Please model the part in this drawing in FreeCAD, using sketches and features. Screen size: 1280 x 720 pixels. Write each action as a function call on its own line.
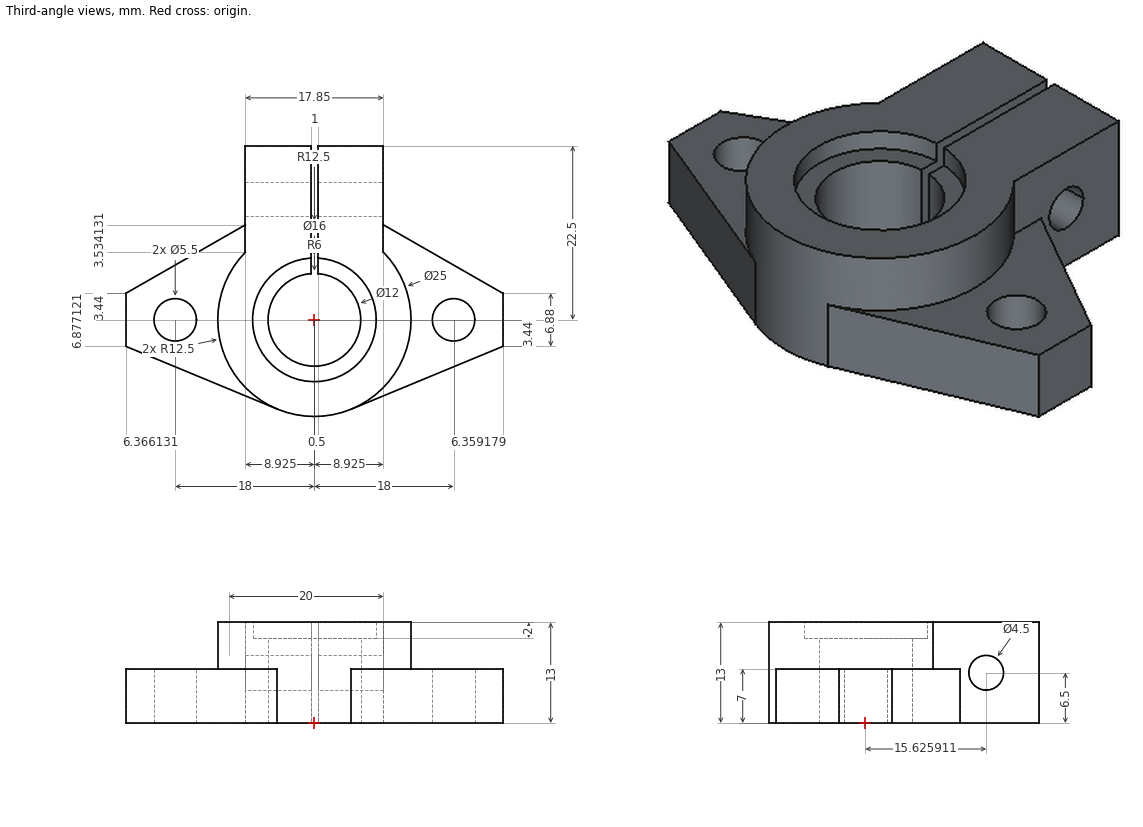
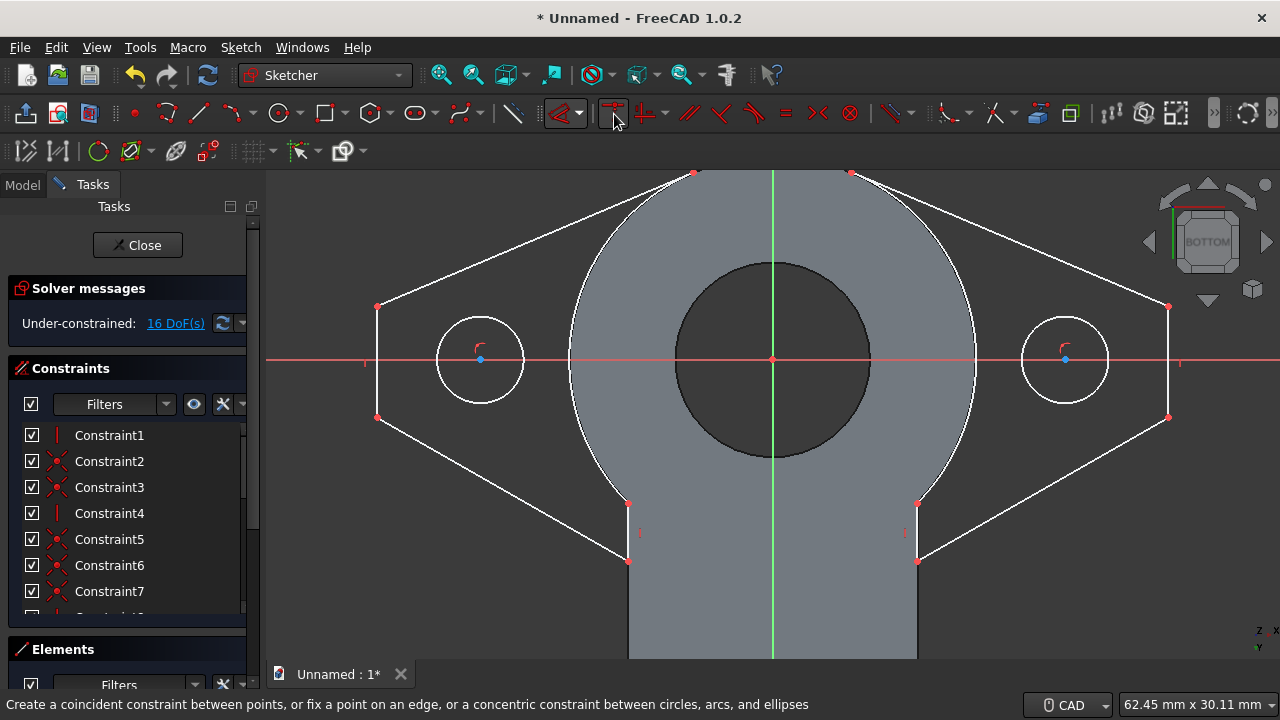
click(603, 247)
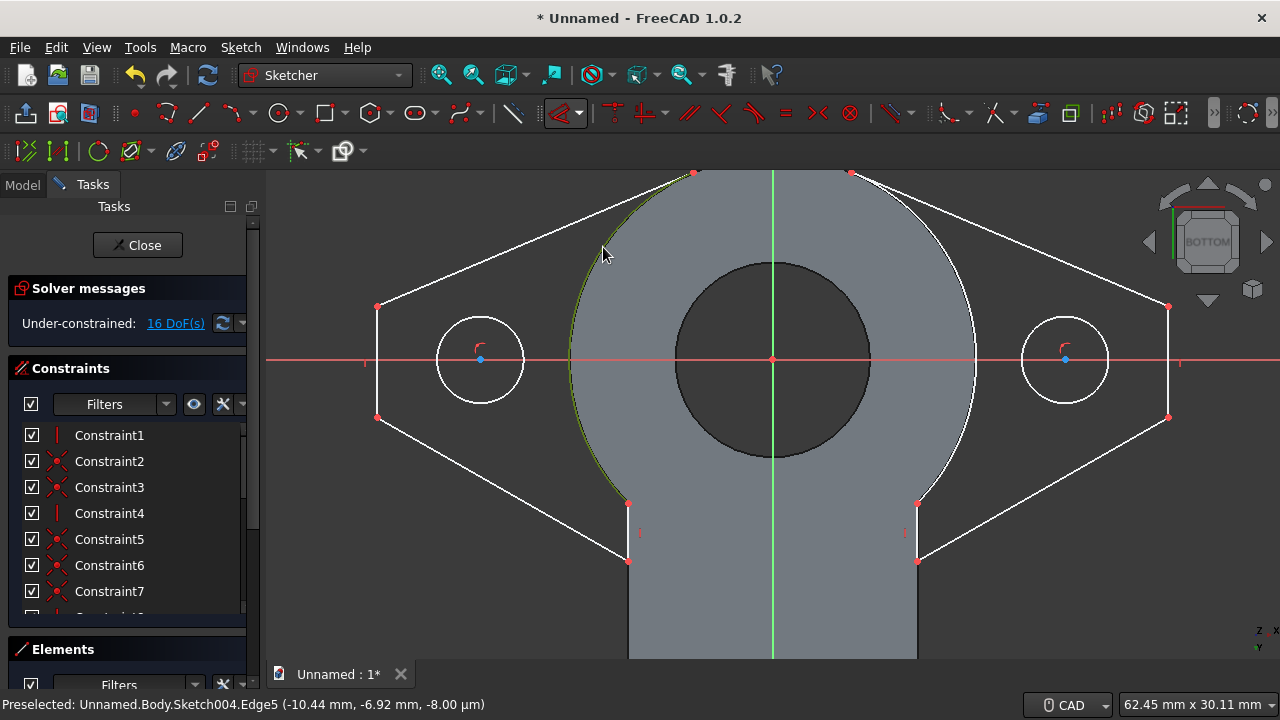
click(972, 399)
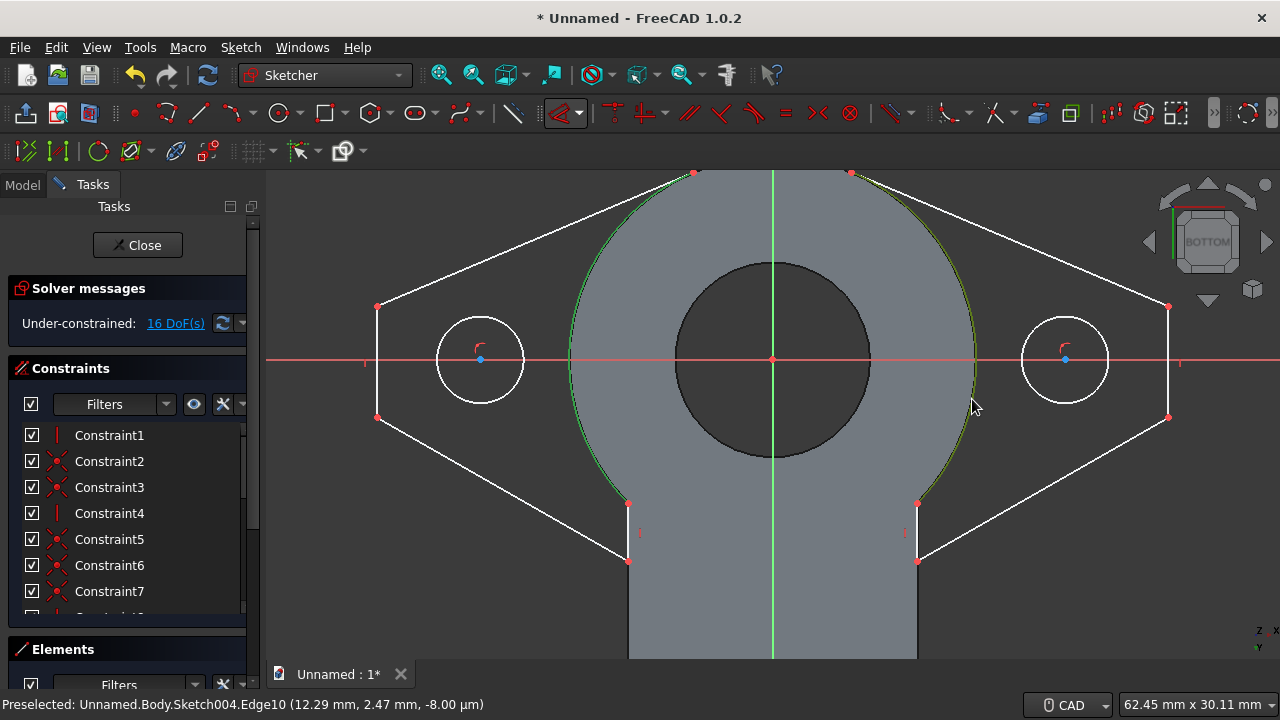
click(786, 114)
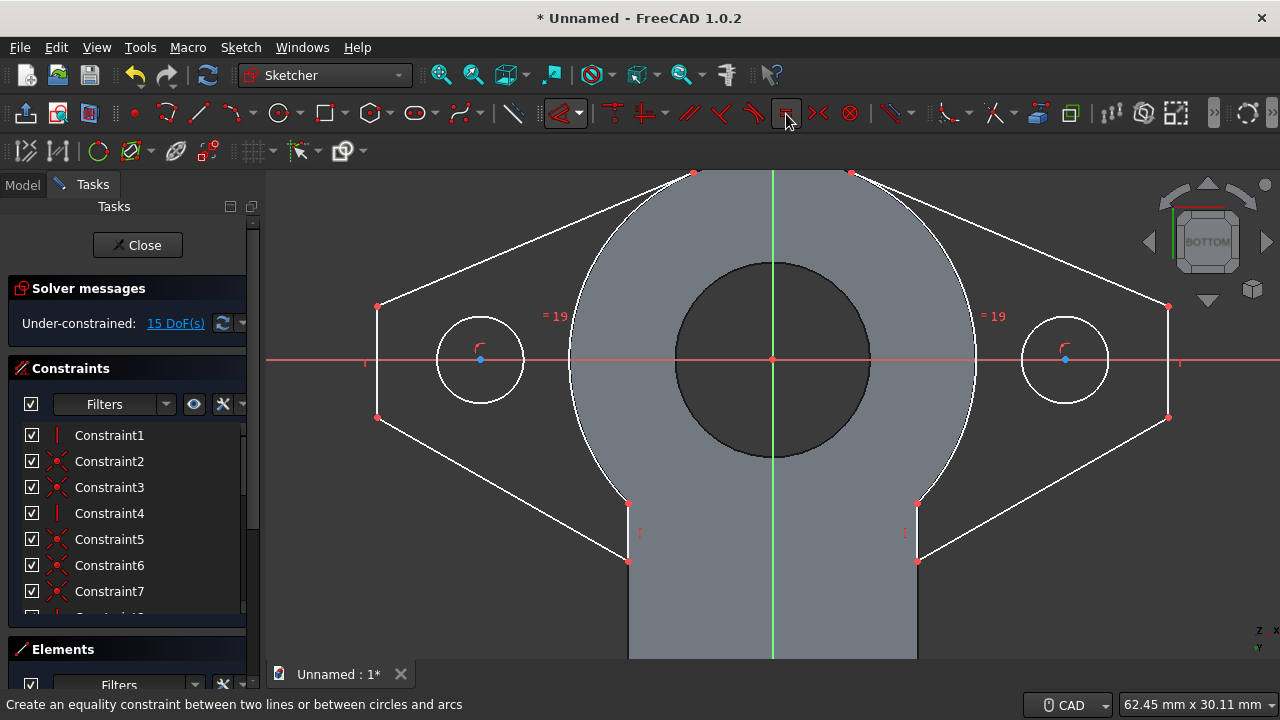
click(511, 329)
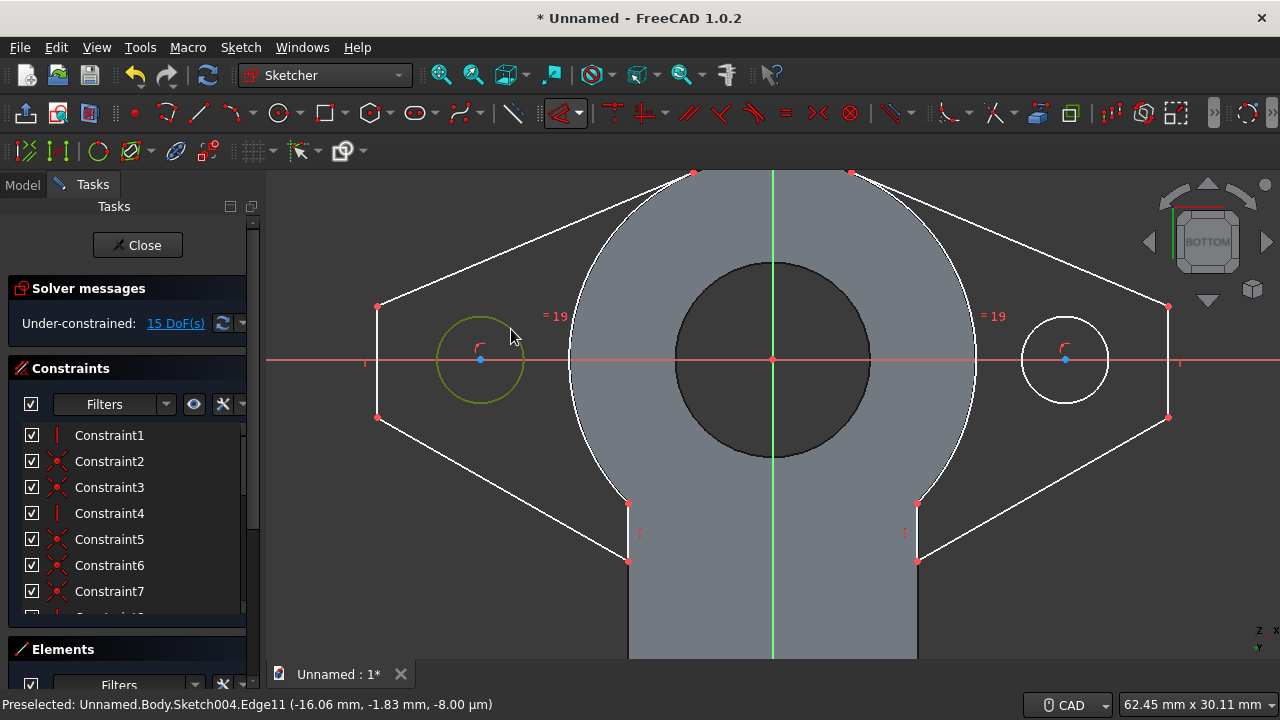
click(1096, 329)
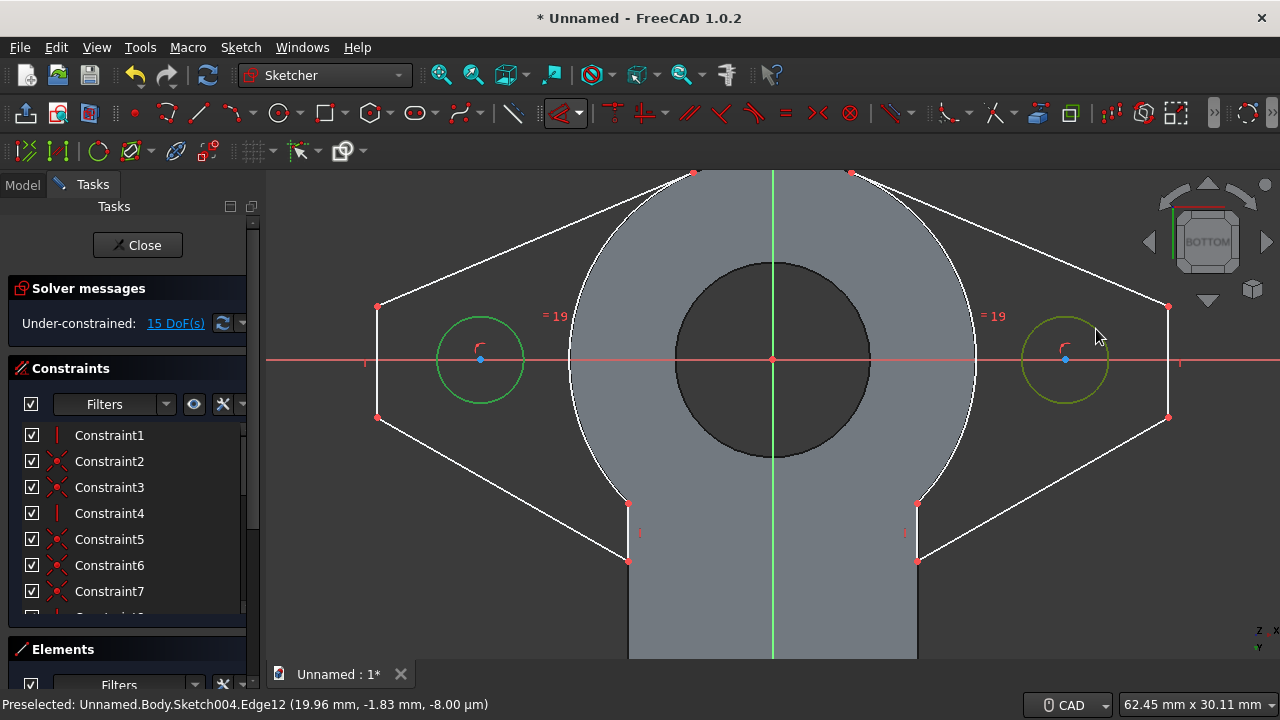
click(786, 114)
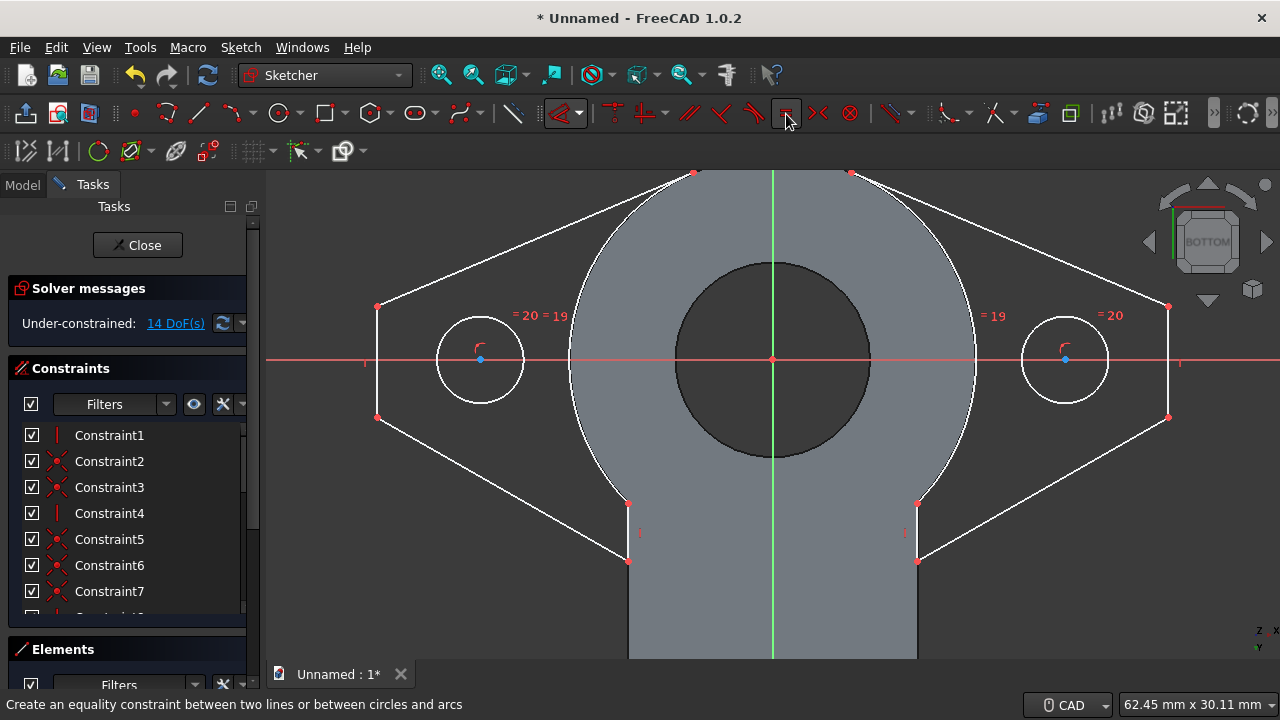
click(603, 247)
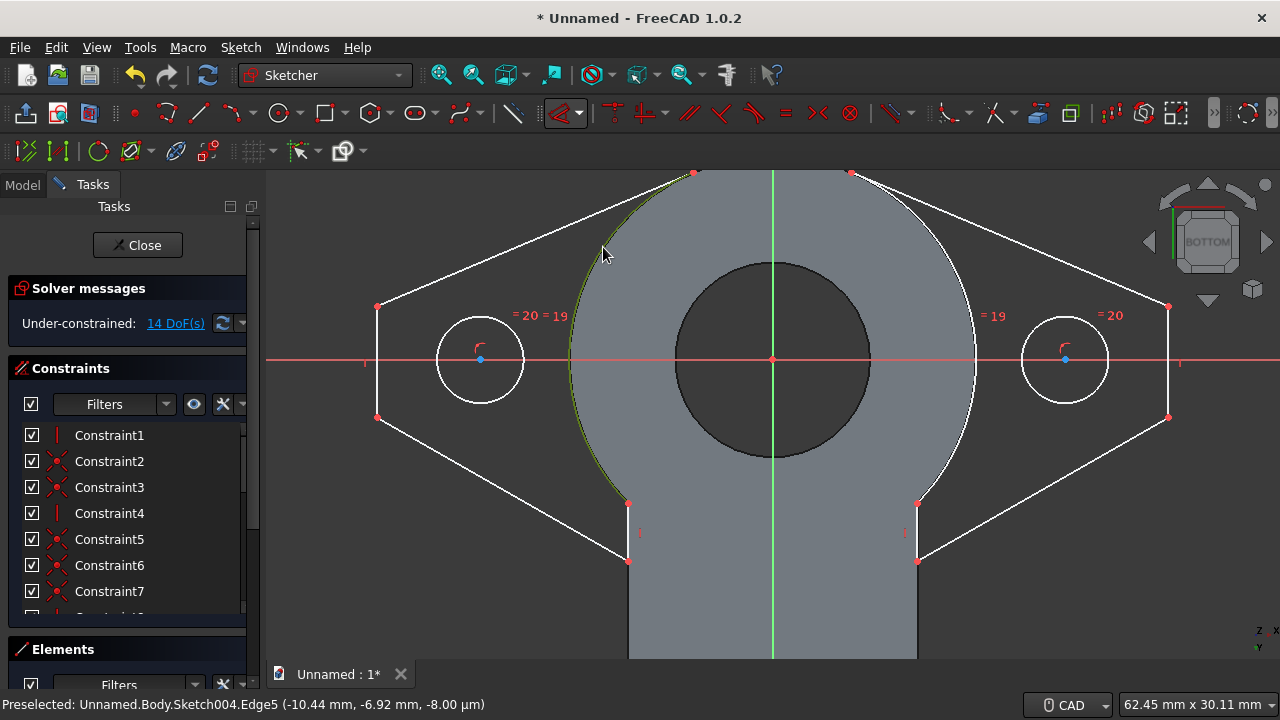
click(582, 114)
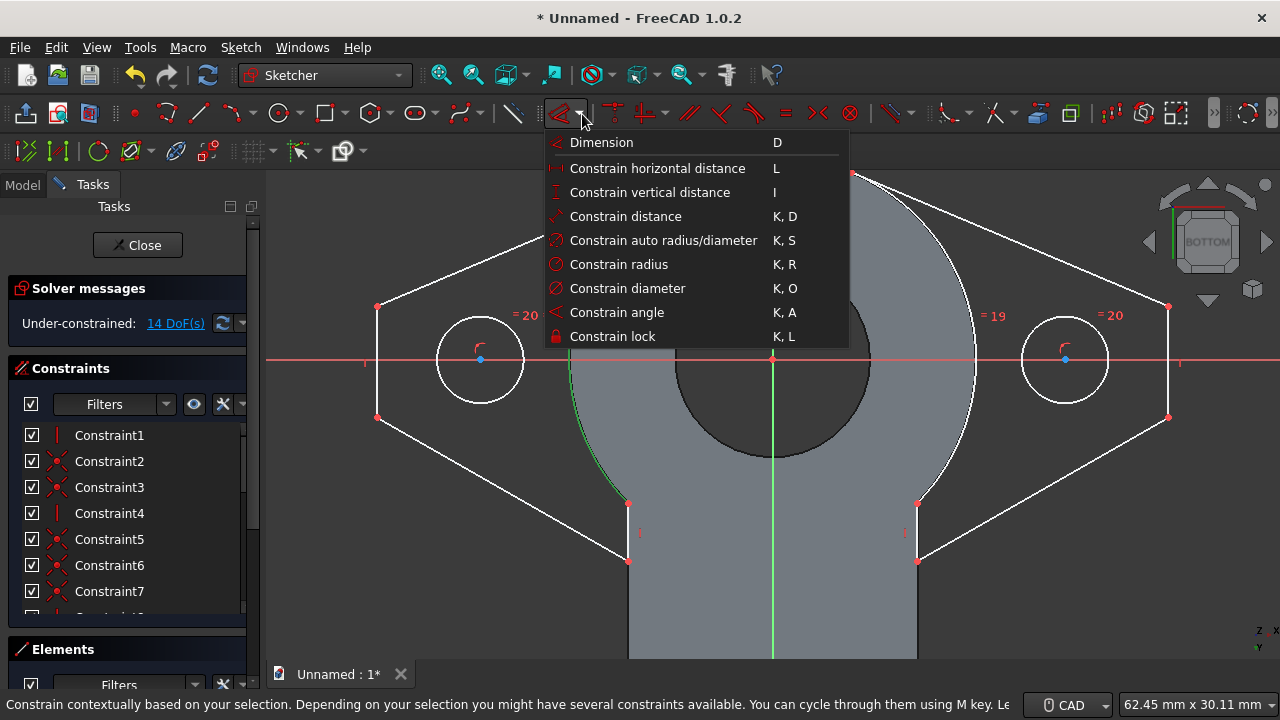
click(697, 264)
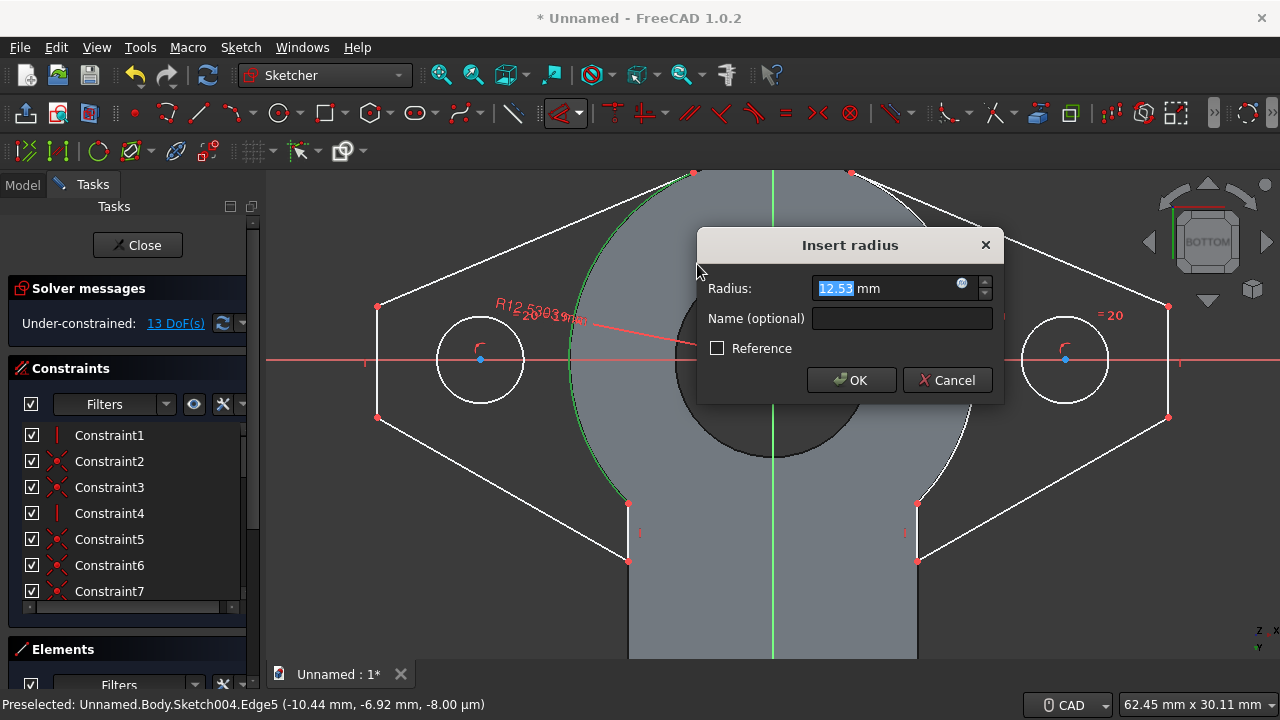
text(12.5)
key(Return)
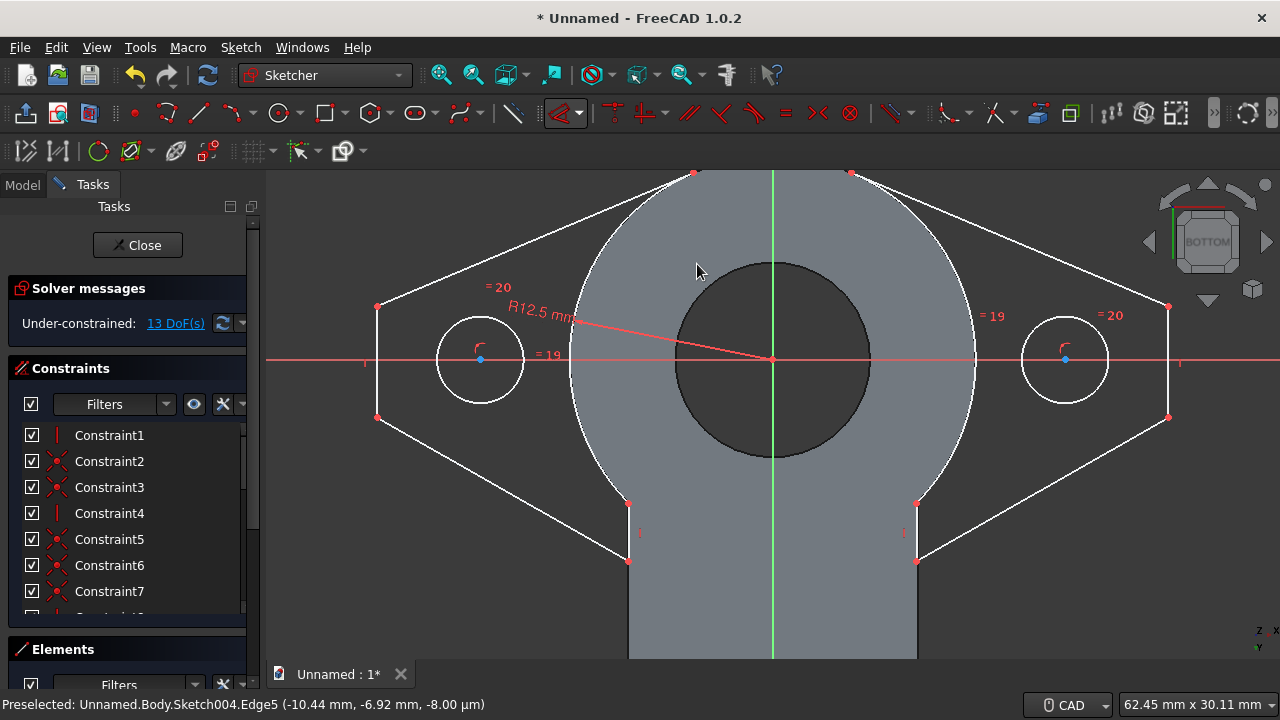
click(511, 329)